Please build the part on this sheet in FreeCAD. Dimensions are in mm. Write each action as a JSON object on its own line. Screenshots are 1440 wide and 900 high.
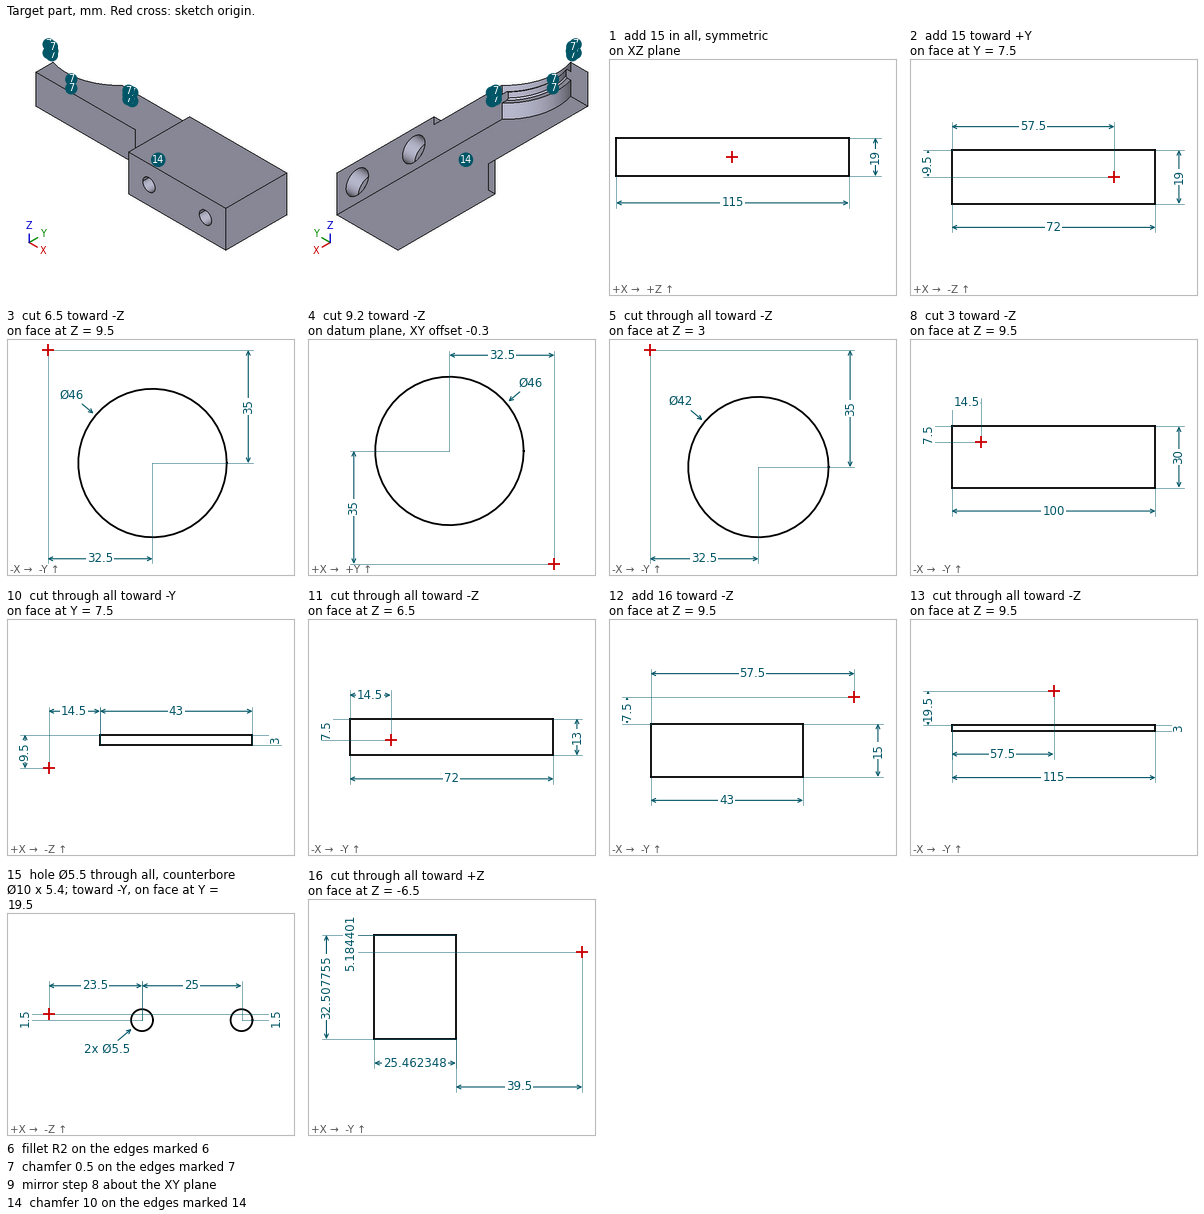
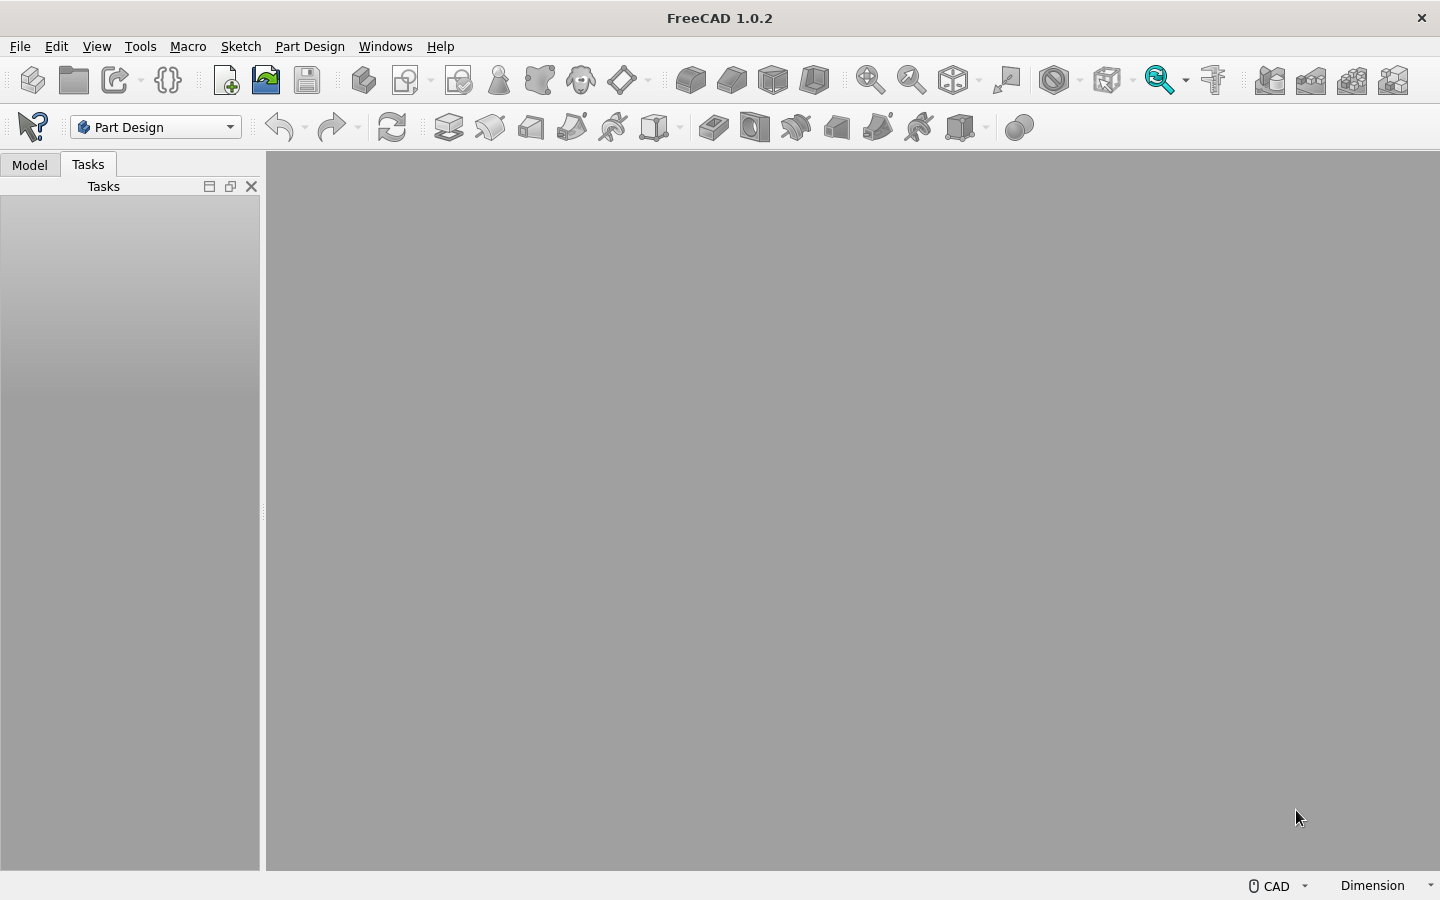
{"action": "left_click", "coordinate": [225, 80]}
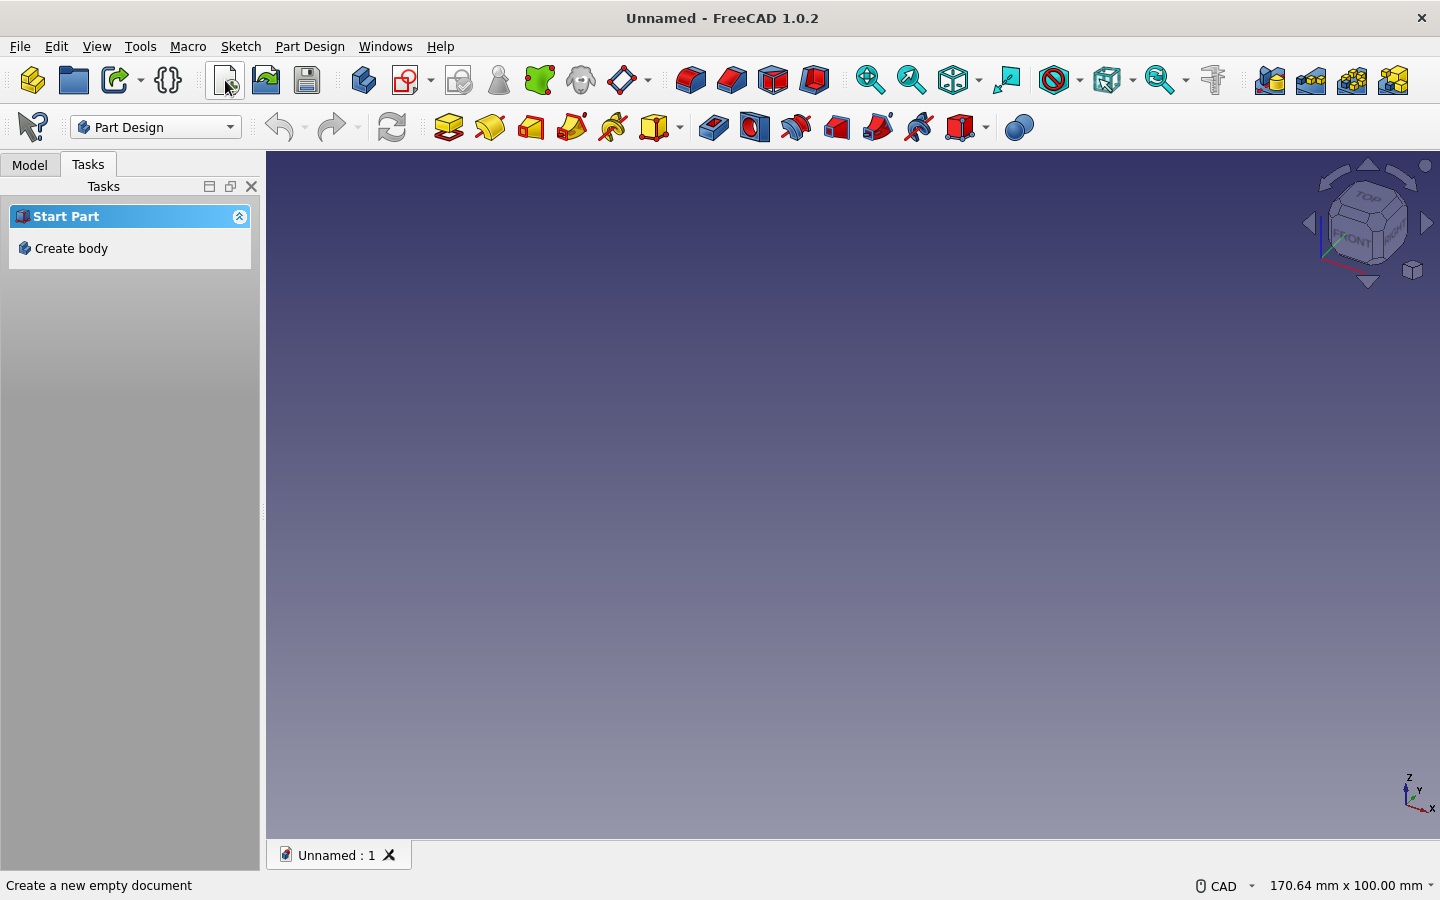
{"action": "left_click", "coordinate": [404, 80]}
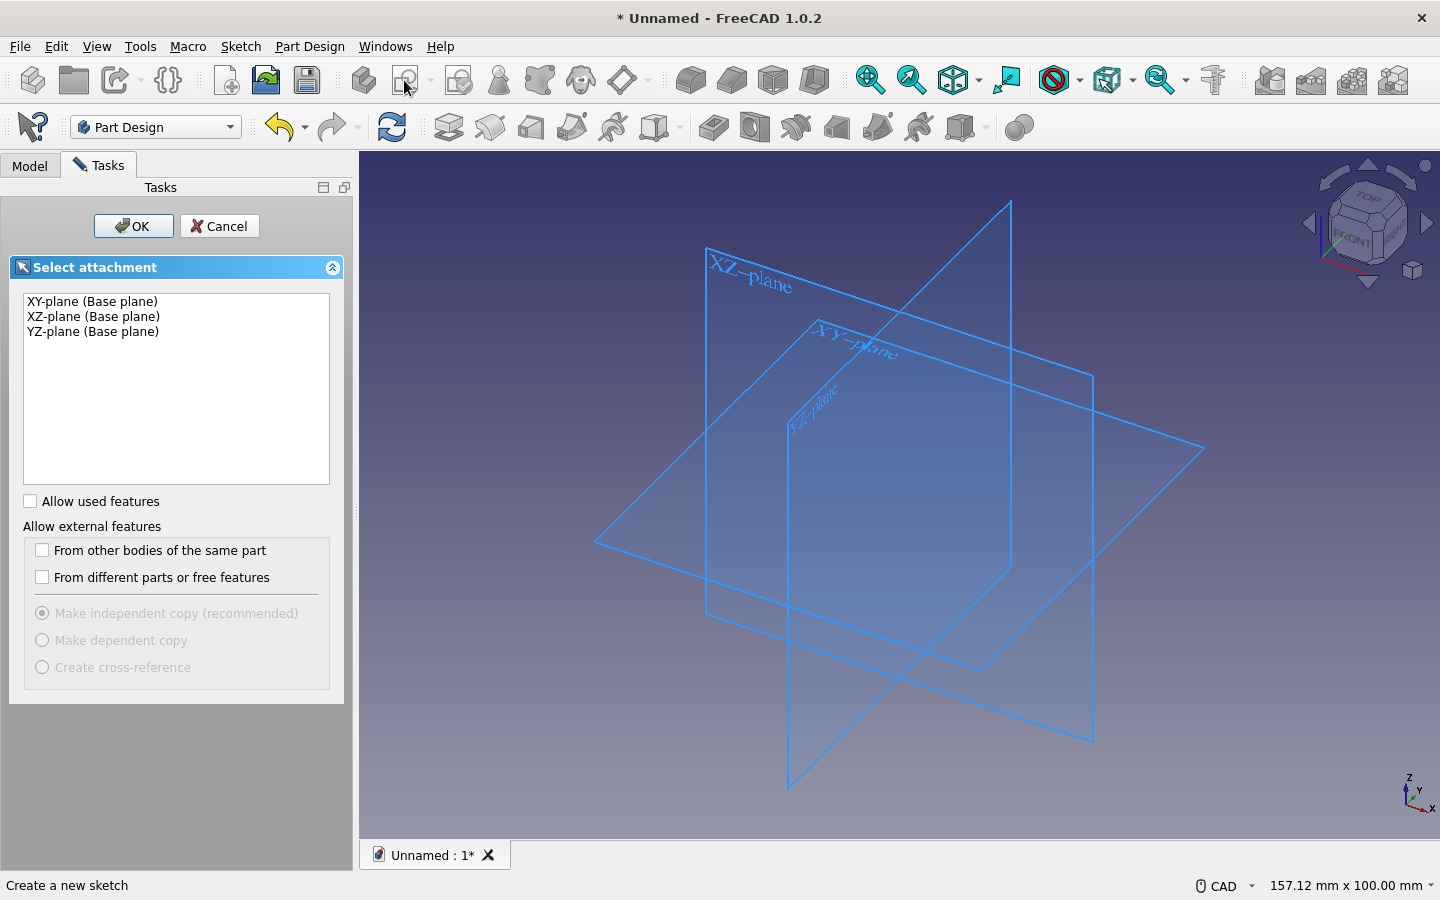
{"action": "left_click", "coordinate": [84, 316]}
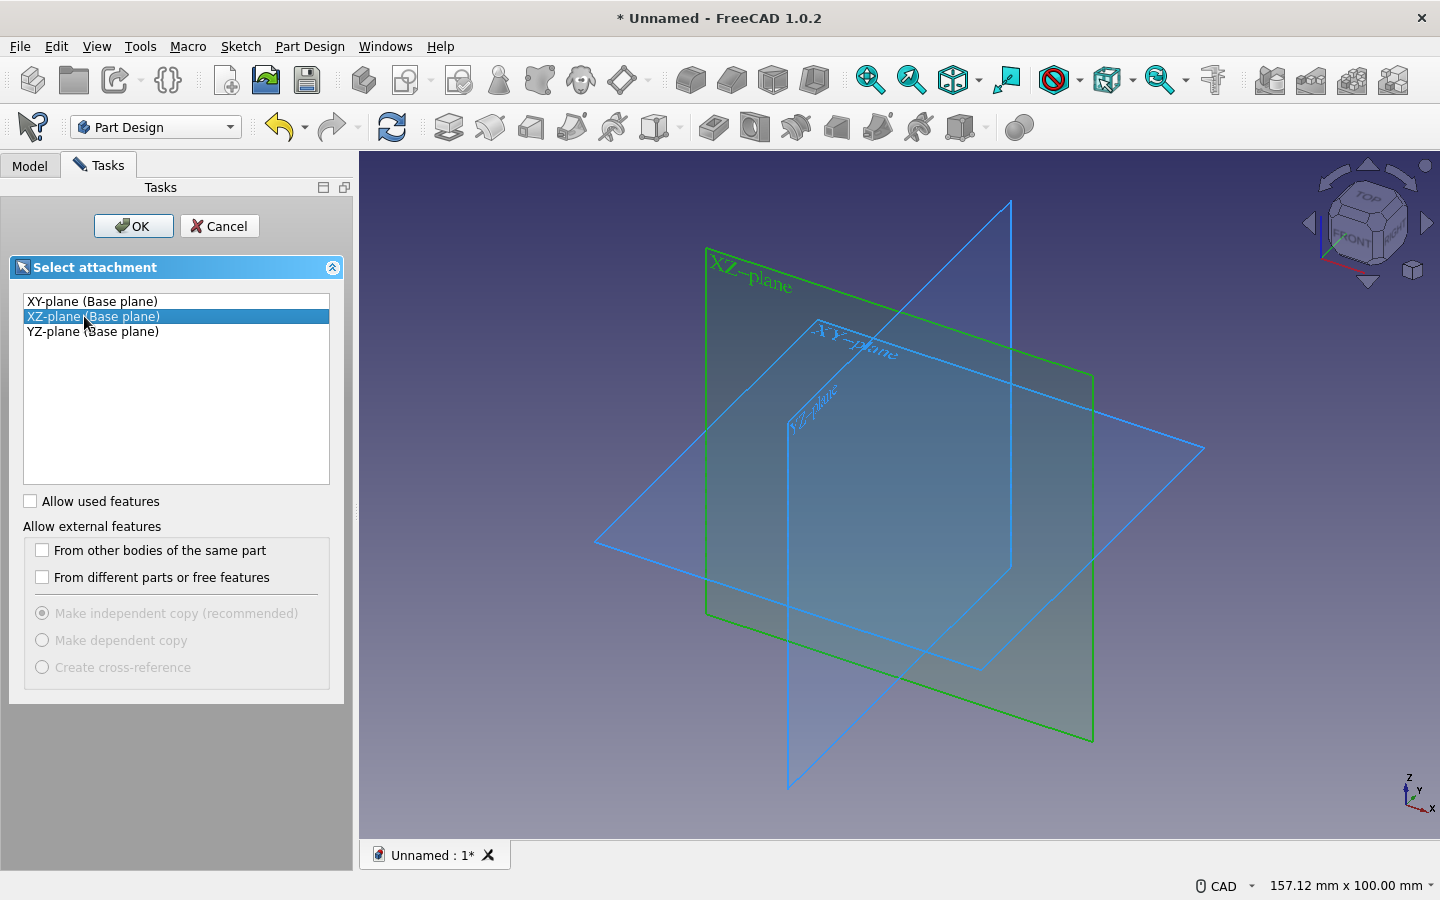
{"action": "left_click", "coordinate": [134, 226]}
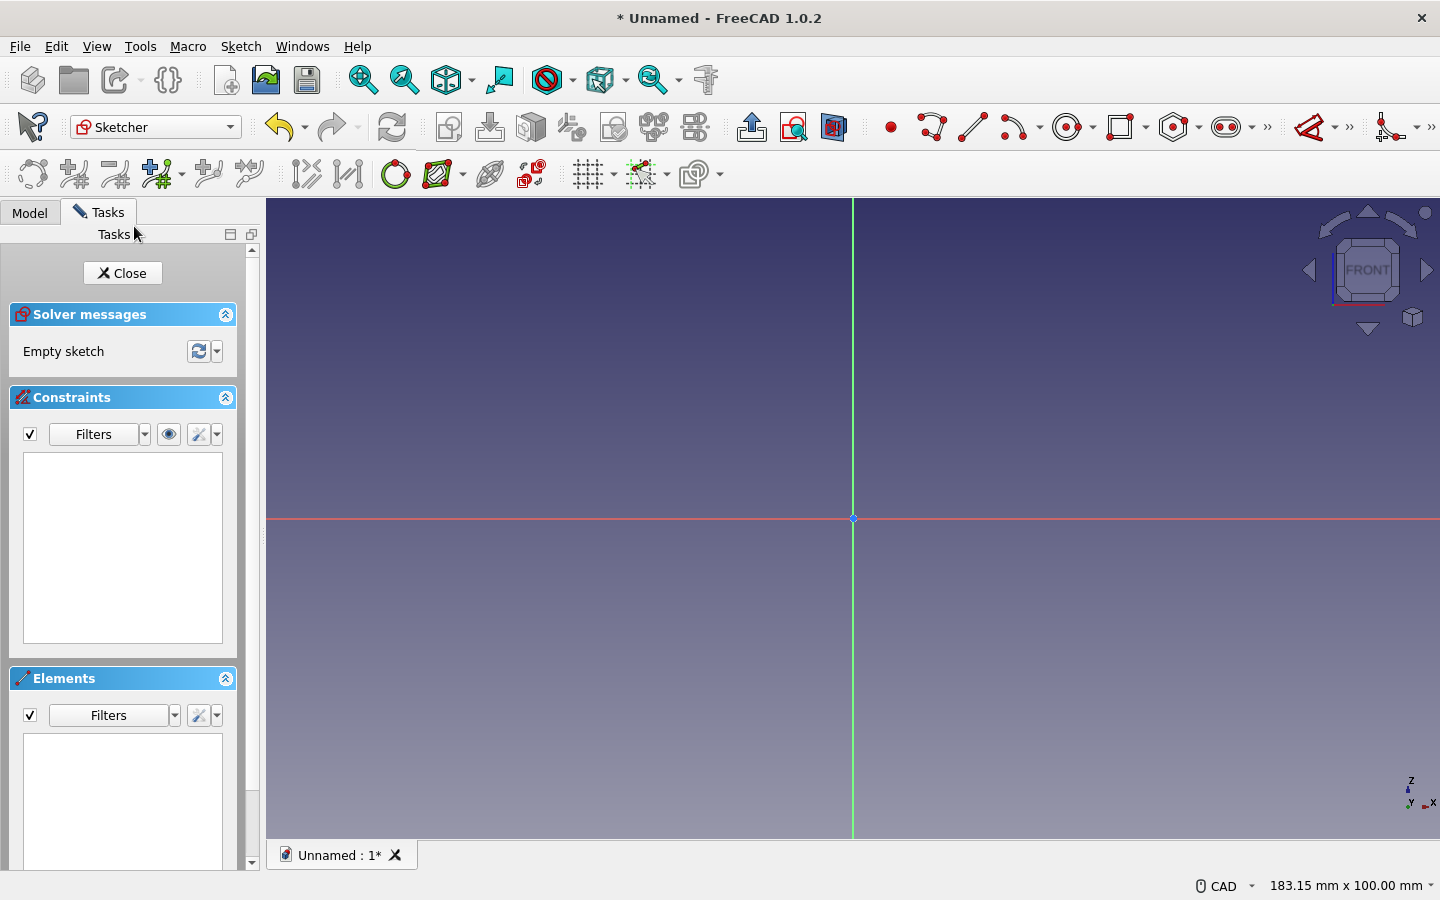
{"action": "key", "text": "g v"}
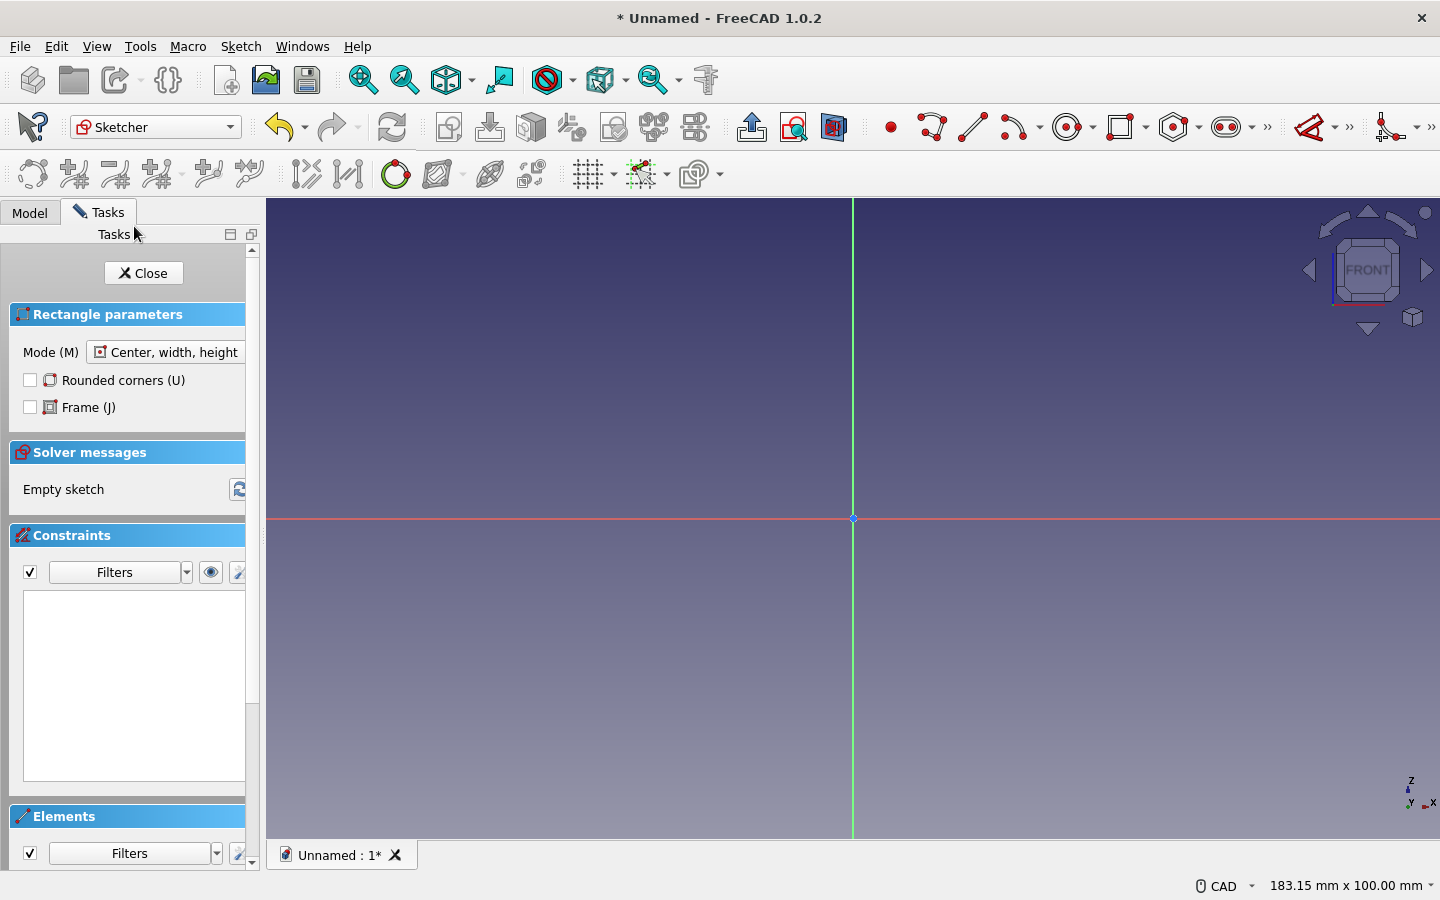
{"action": "left_click", "coordinate": [853, 518]}
{"action": "mouse_move", "coordinate": [1222, 458]}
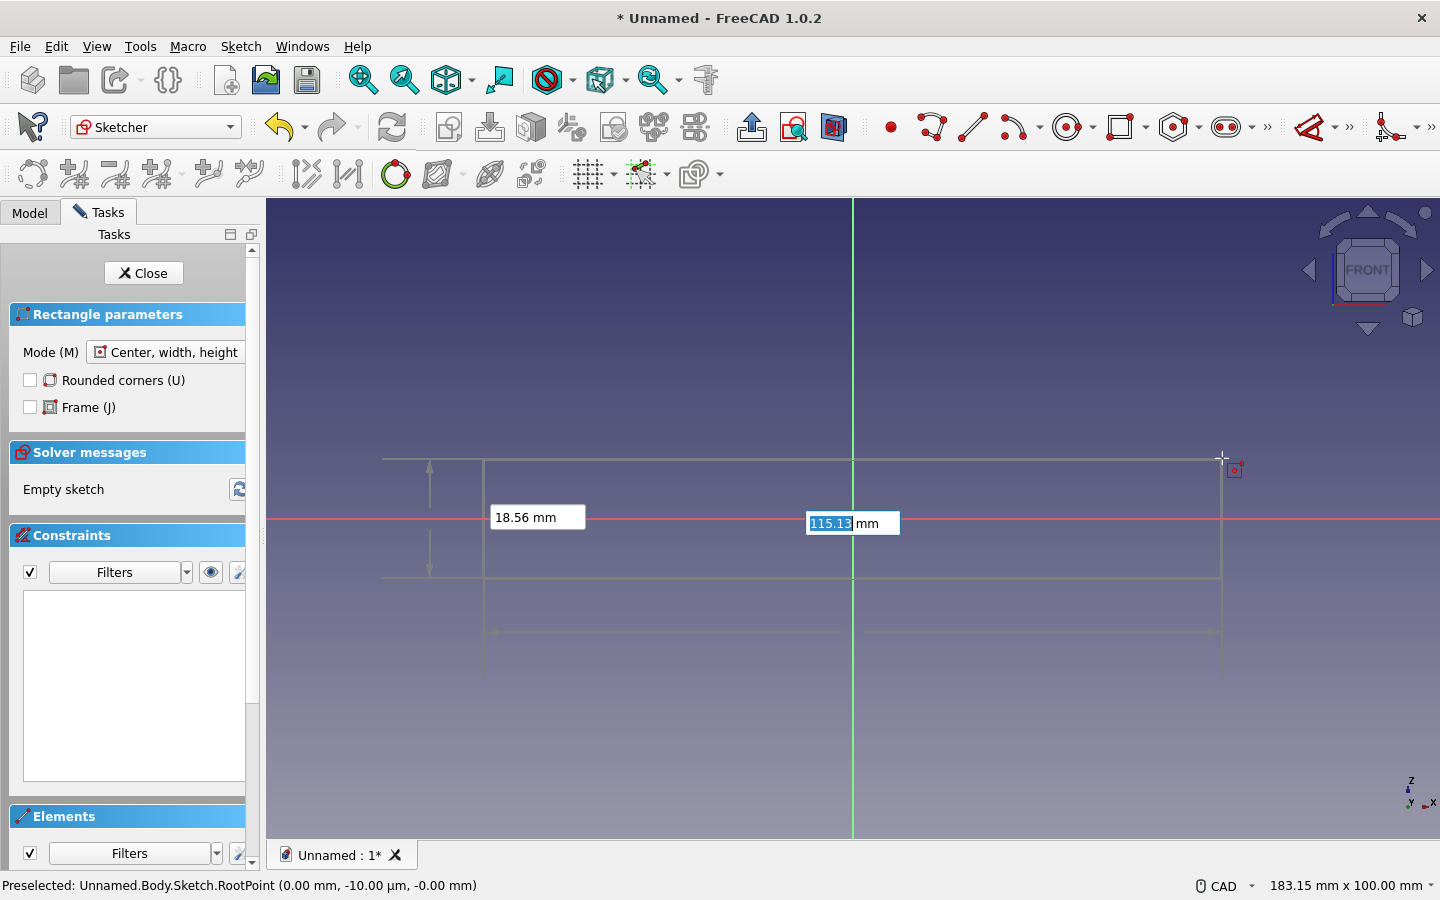
{"action": "type", "text": "115"}
{"action": "key", "text": "Tab"}
{"action": "type", "text": "19"}
{"action": "key", "text": "Return"}
{"action": "key", "text": "Escape"}